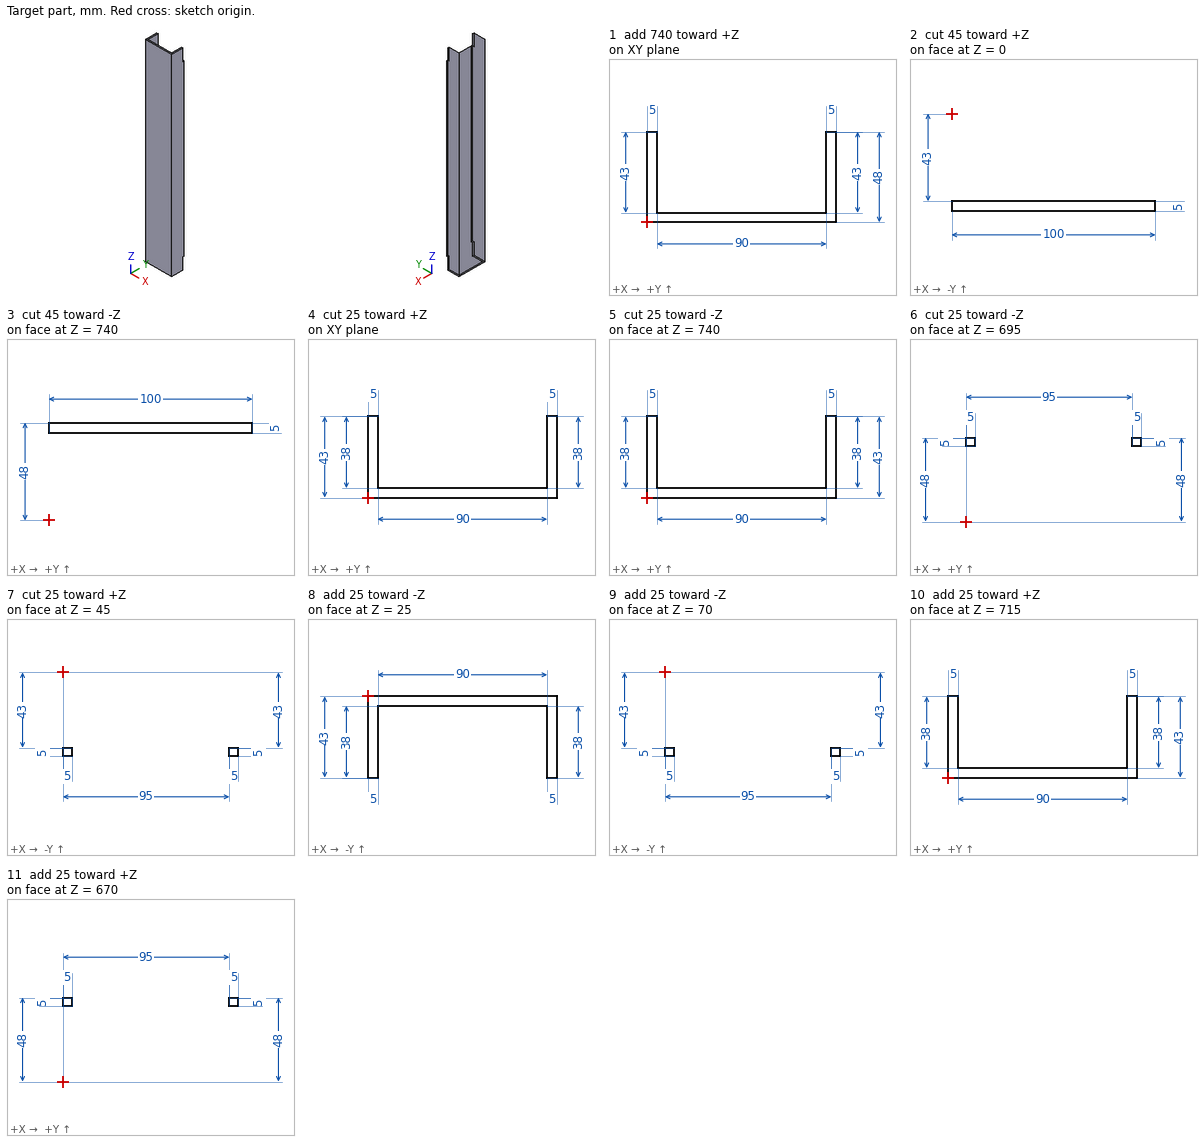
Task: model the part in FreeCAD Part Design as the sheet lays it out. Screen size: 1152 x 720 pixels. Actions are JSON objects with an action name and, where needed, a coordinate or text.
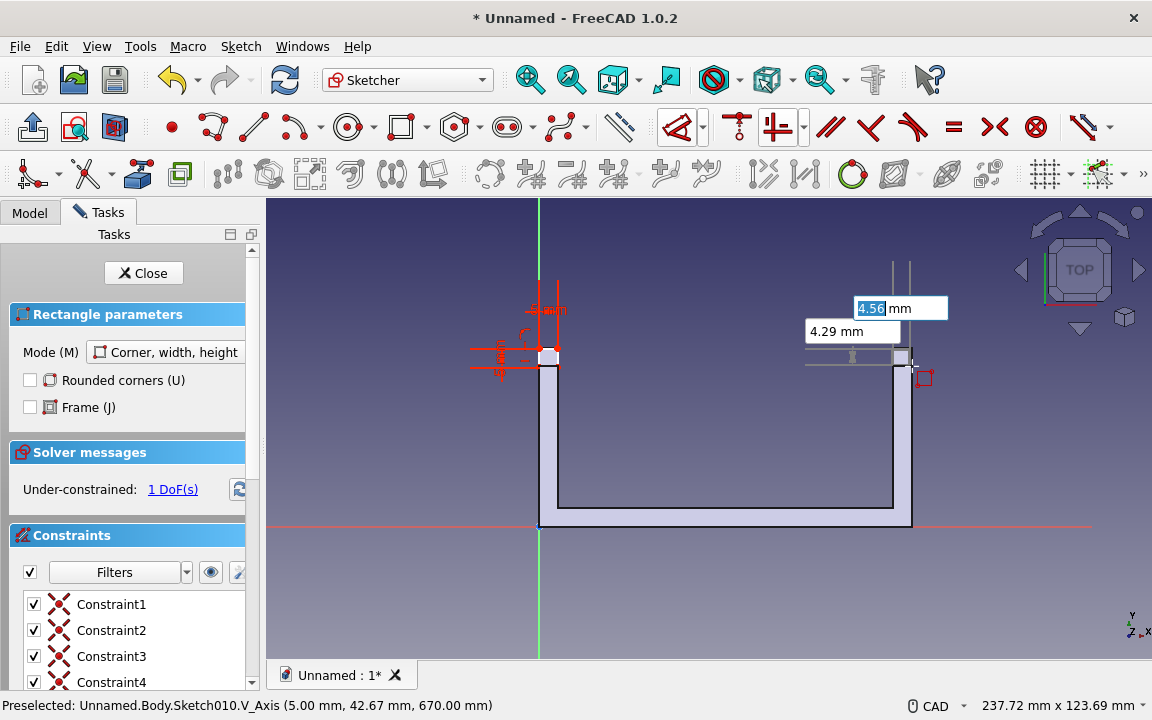
{"action": "type", "text": "5"}
{"action": "key", "text": "Tab"}
{"action": "type", "text": "5"}
{"action": "key", "text": "Return"}
{"action": "key", "text": "Escape"}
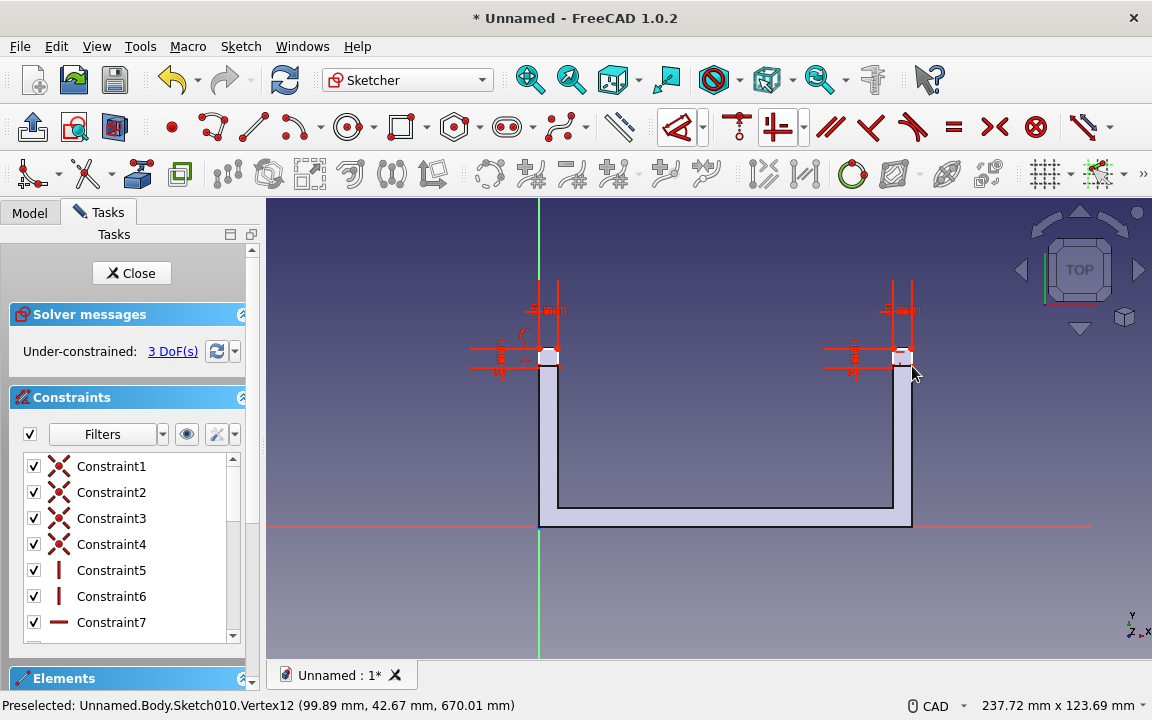
{"action": "left_click", "coordinate": [539, 349]}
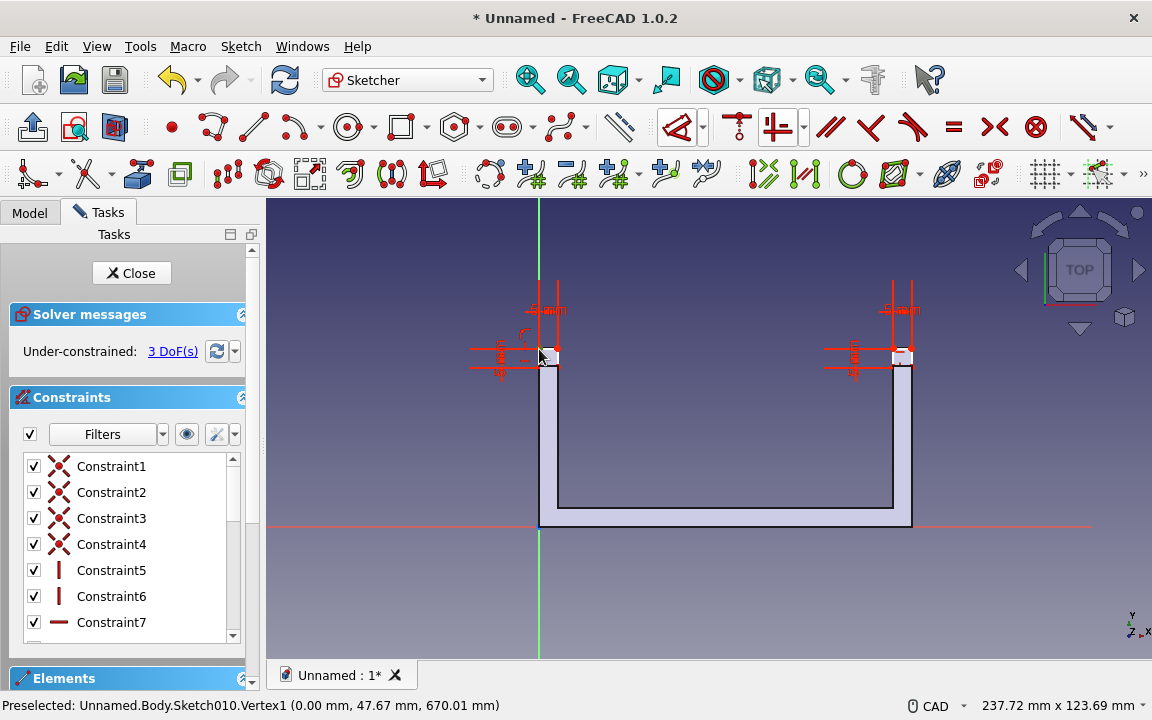
{"action": "key", "text": "i"}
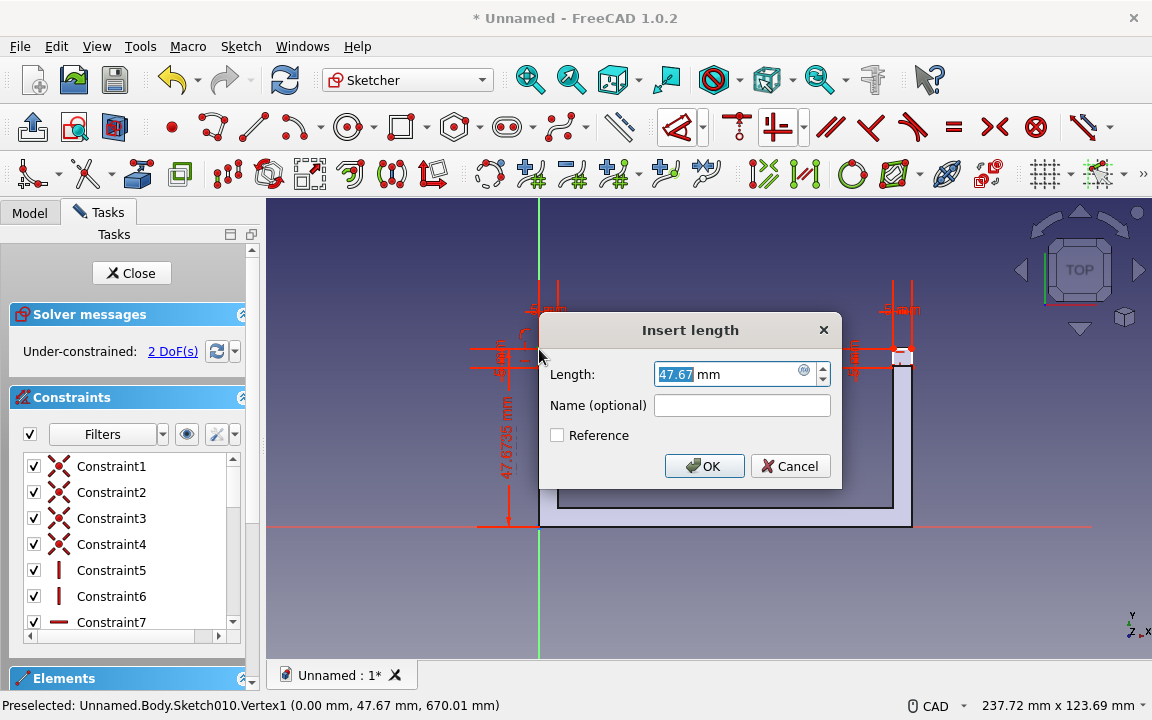
{"action": "type", "text": "48"}
{"action": "key", "text": "Return"}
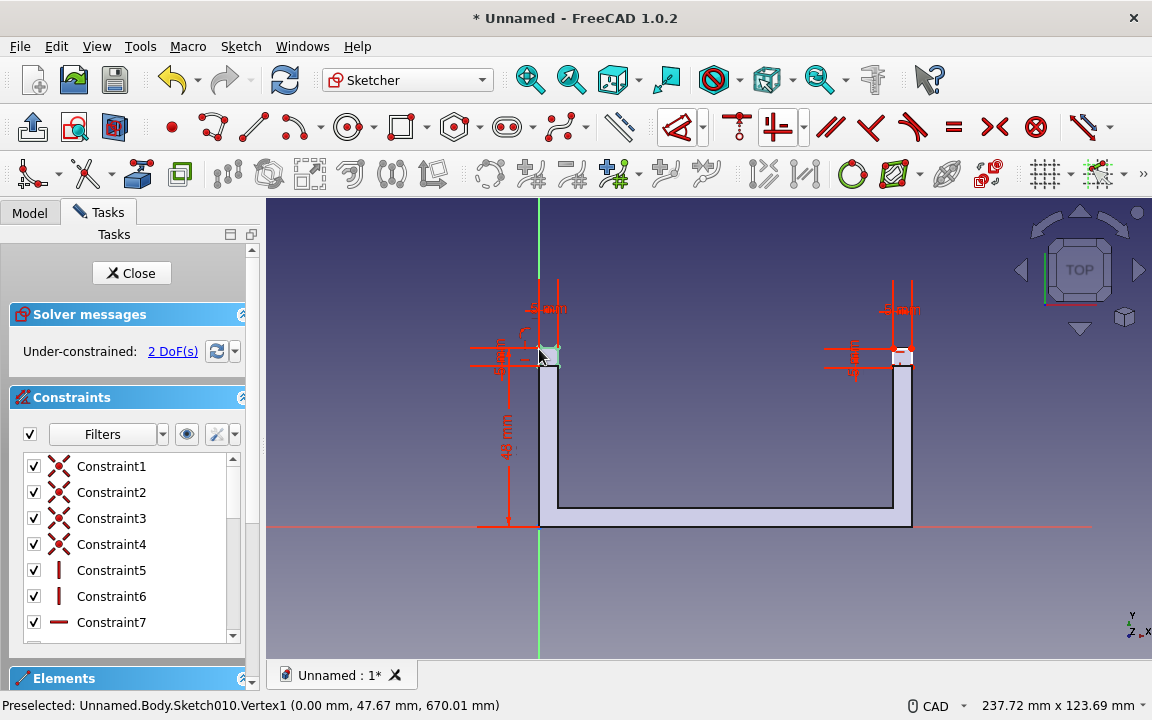
{"action": "left_click", "coordinate": [893, 349]}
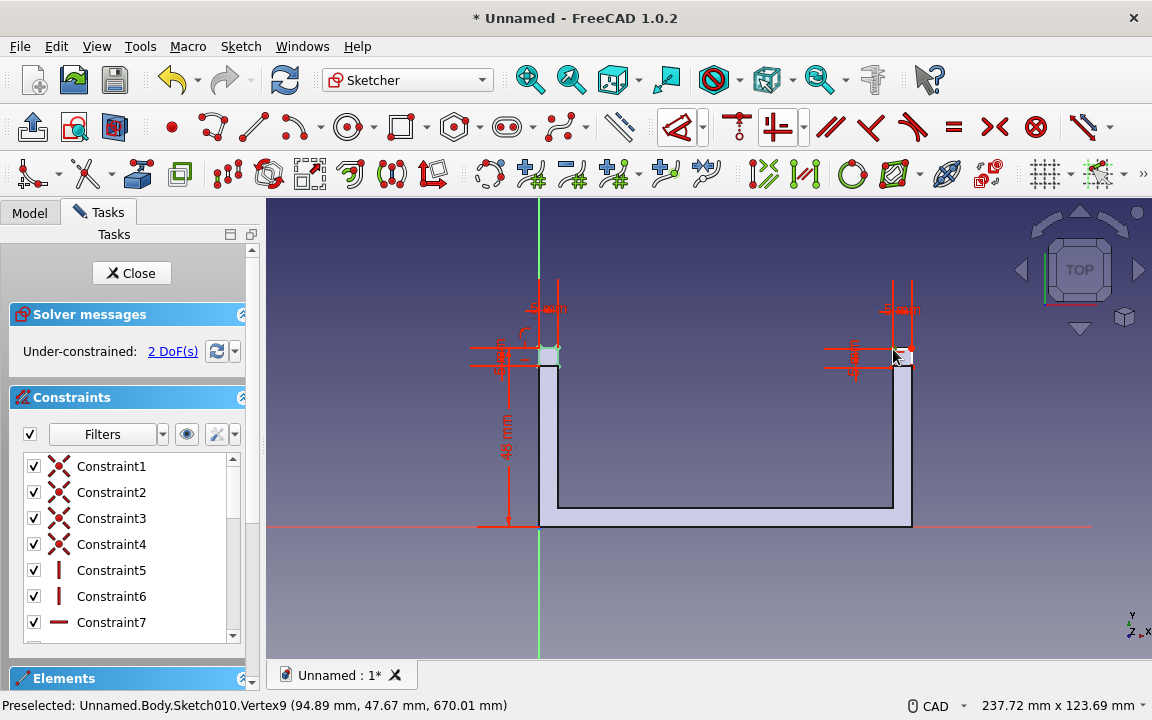
{"action": "key", "text": "l"}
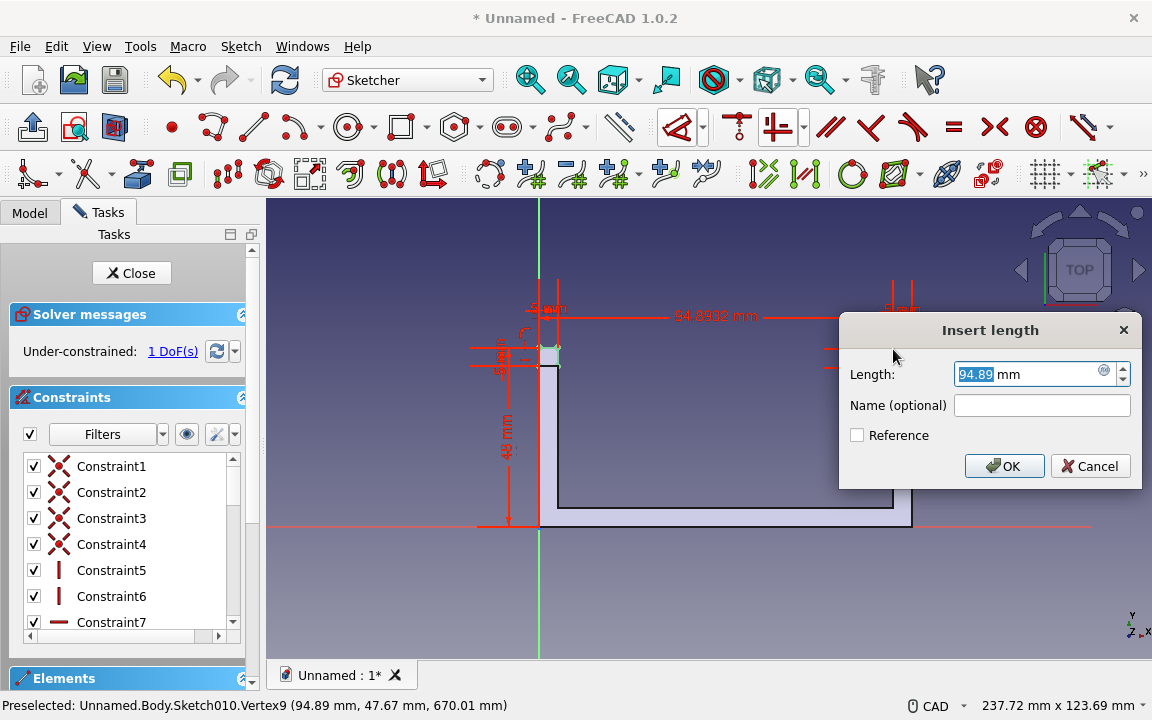
{"action": "type", "text": "95"}
{"action": "key", "text": "Return"}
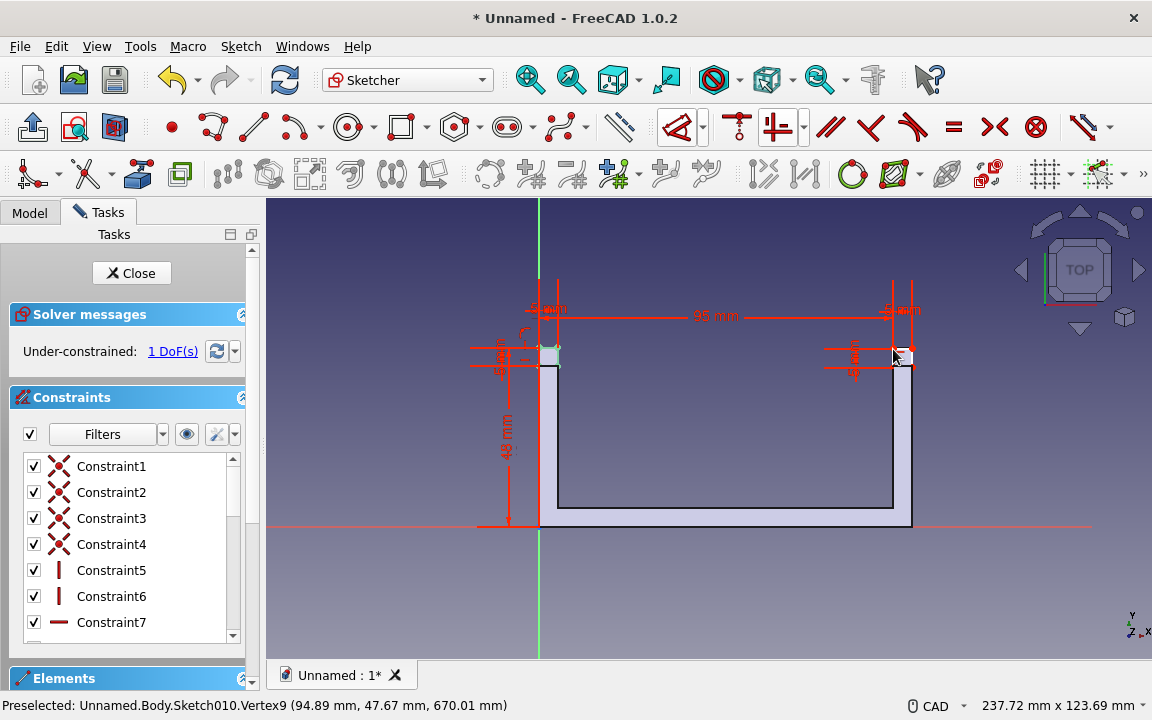
{"action": "left_click", "coordinate": [893, 349]}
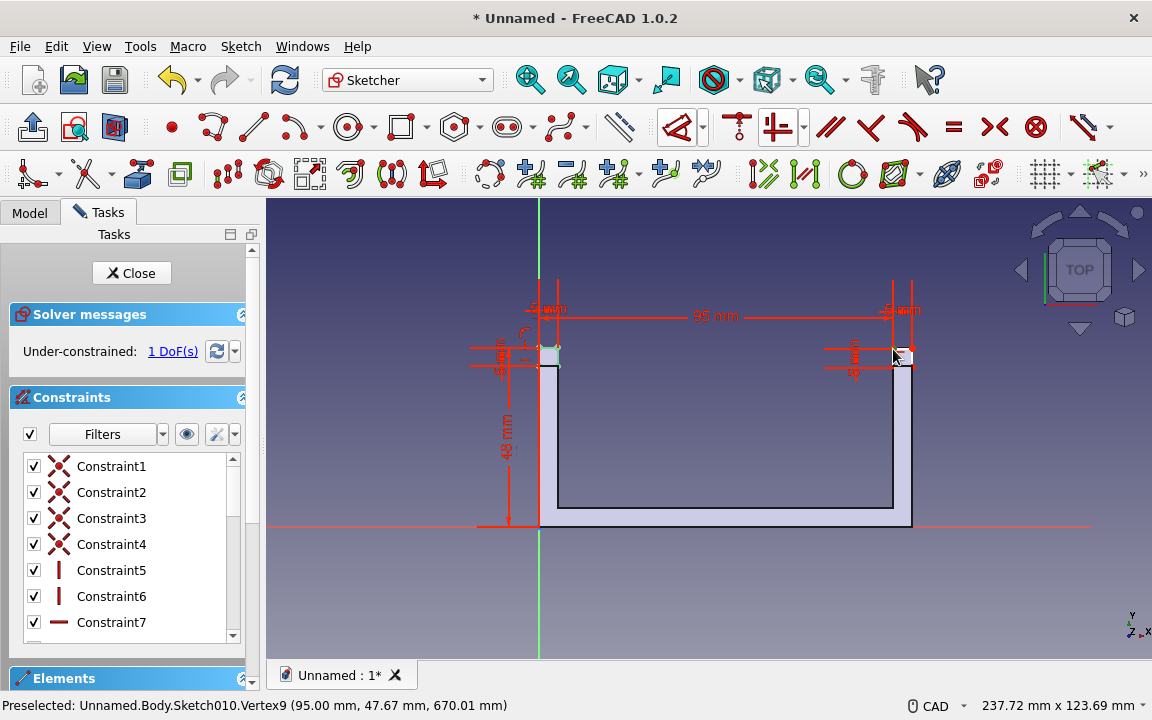
{"action": "key", "text": "i"}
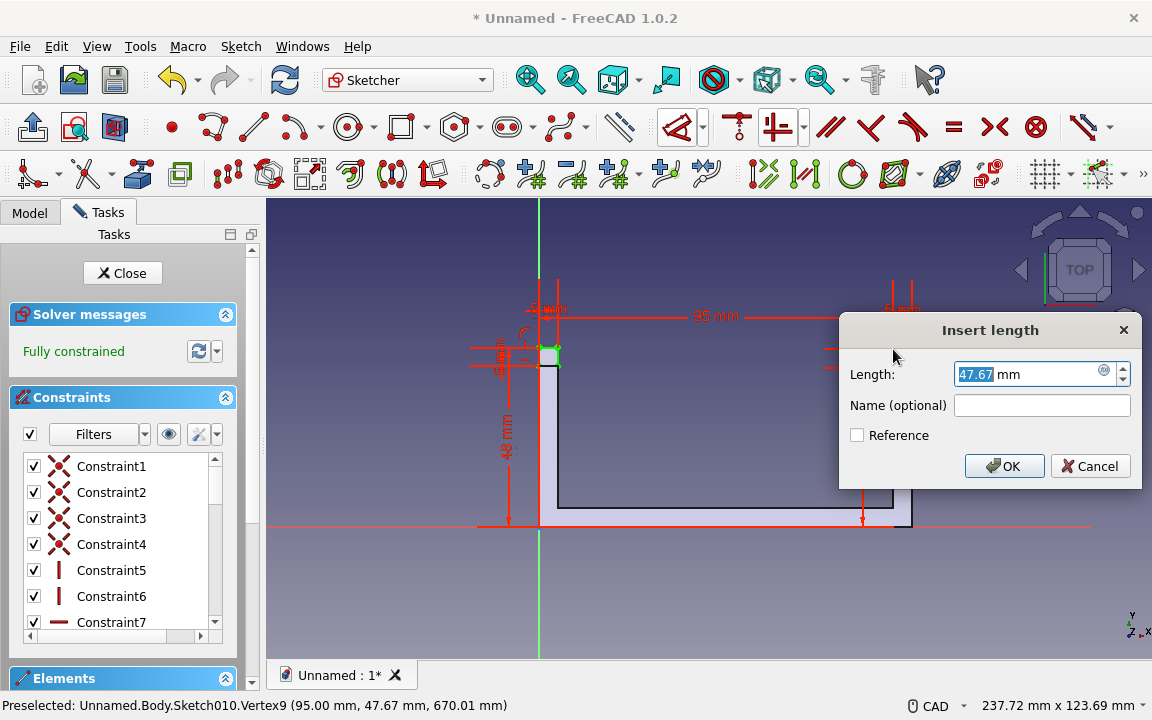
{"action": "type", "text": "48"}
{"action": "key", "text": "Return"}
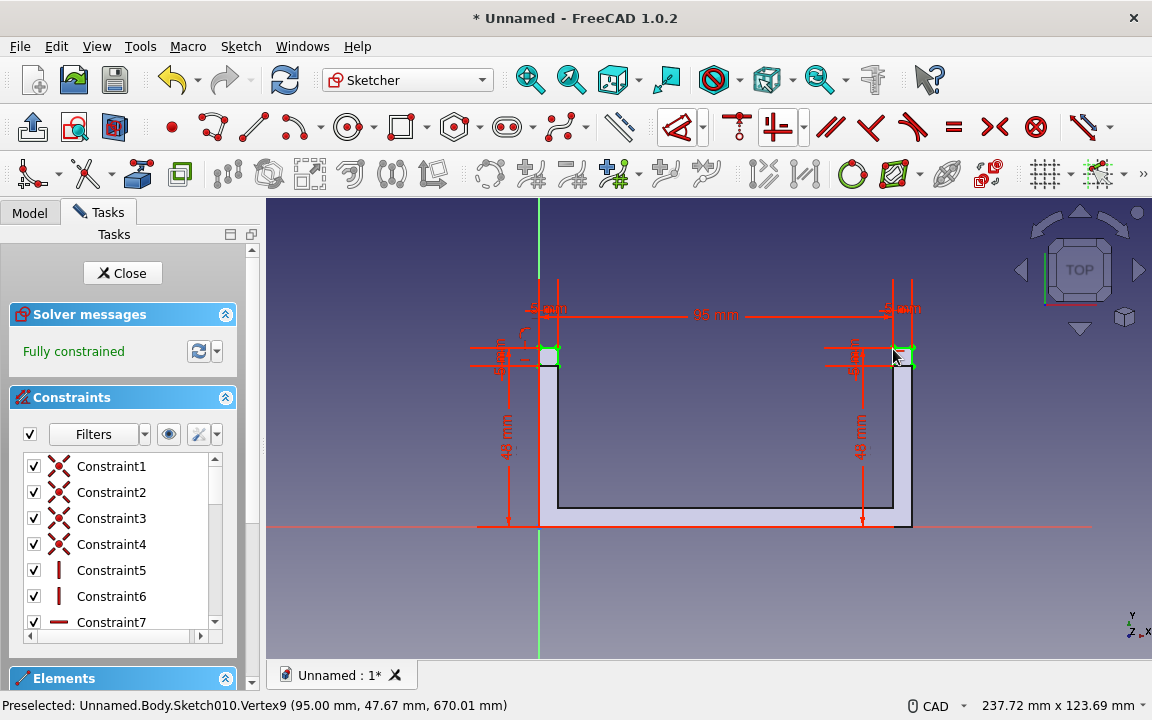
{"action": "left_click", "coordinate": [123, 273]}